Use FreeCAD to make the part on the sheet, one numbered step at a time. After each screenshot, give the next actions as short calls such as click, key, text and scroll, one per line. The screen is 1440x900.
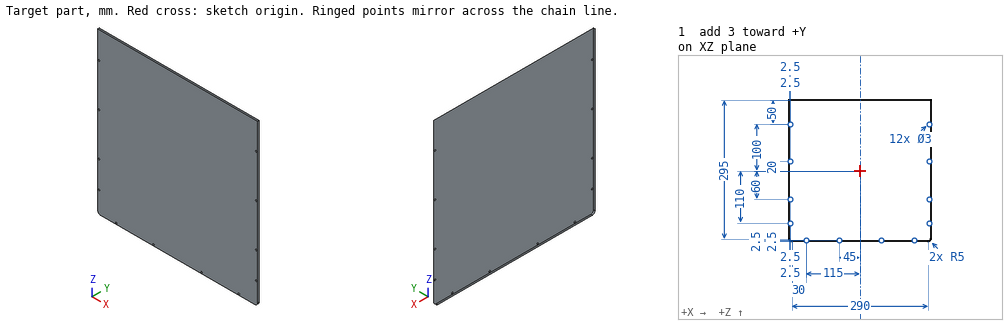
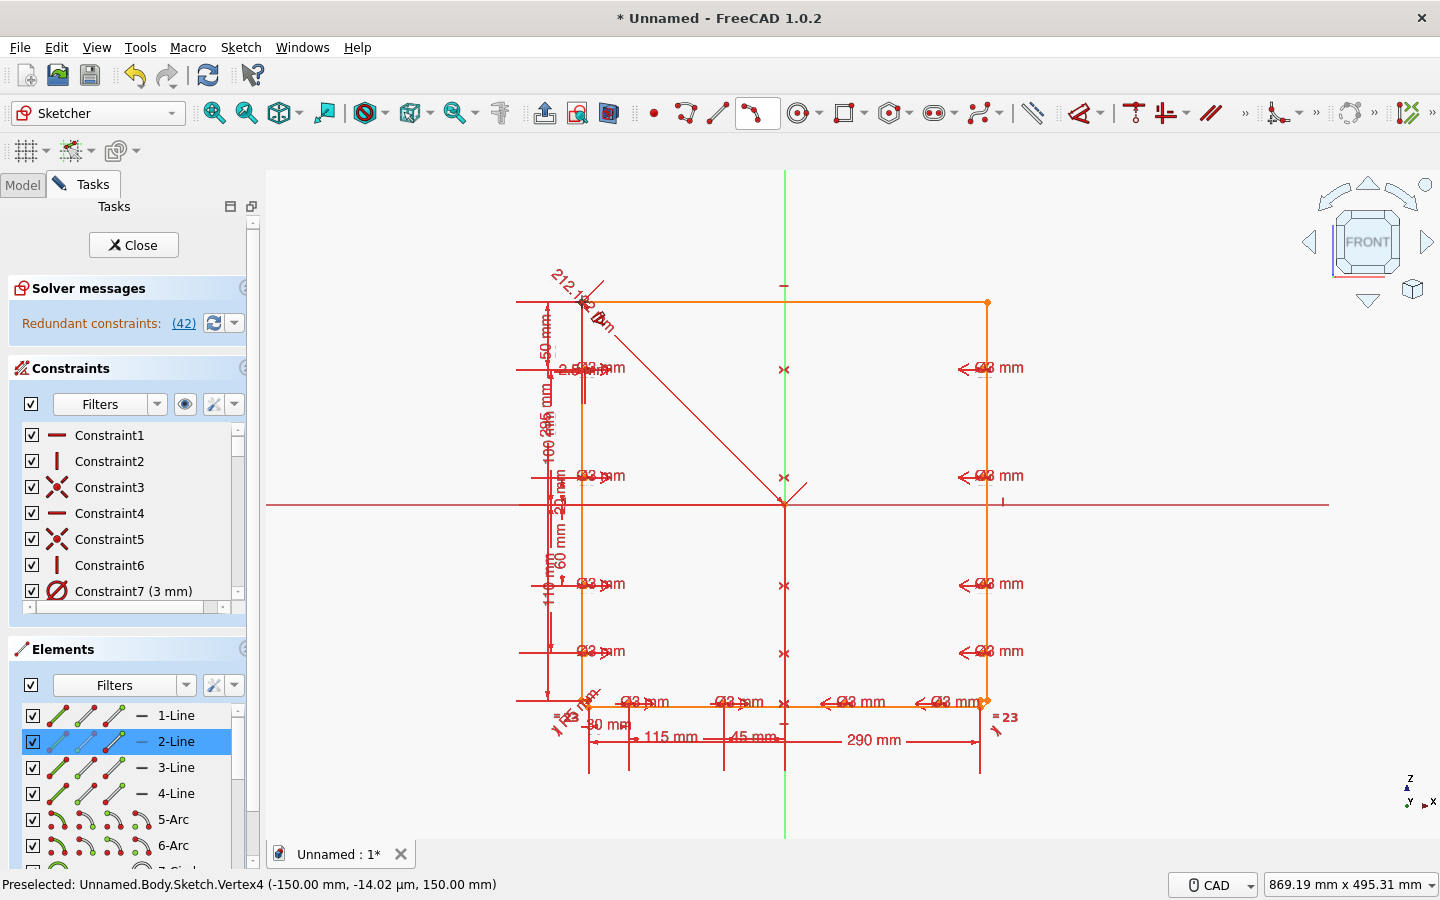
scroll(585, 478, up, 13)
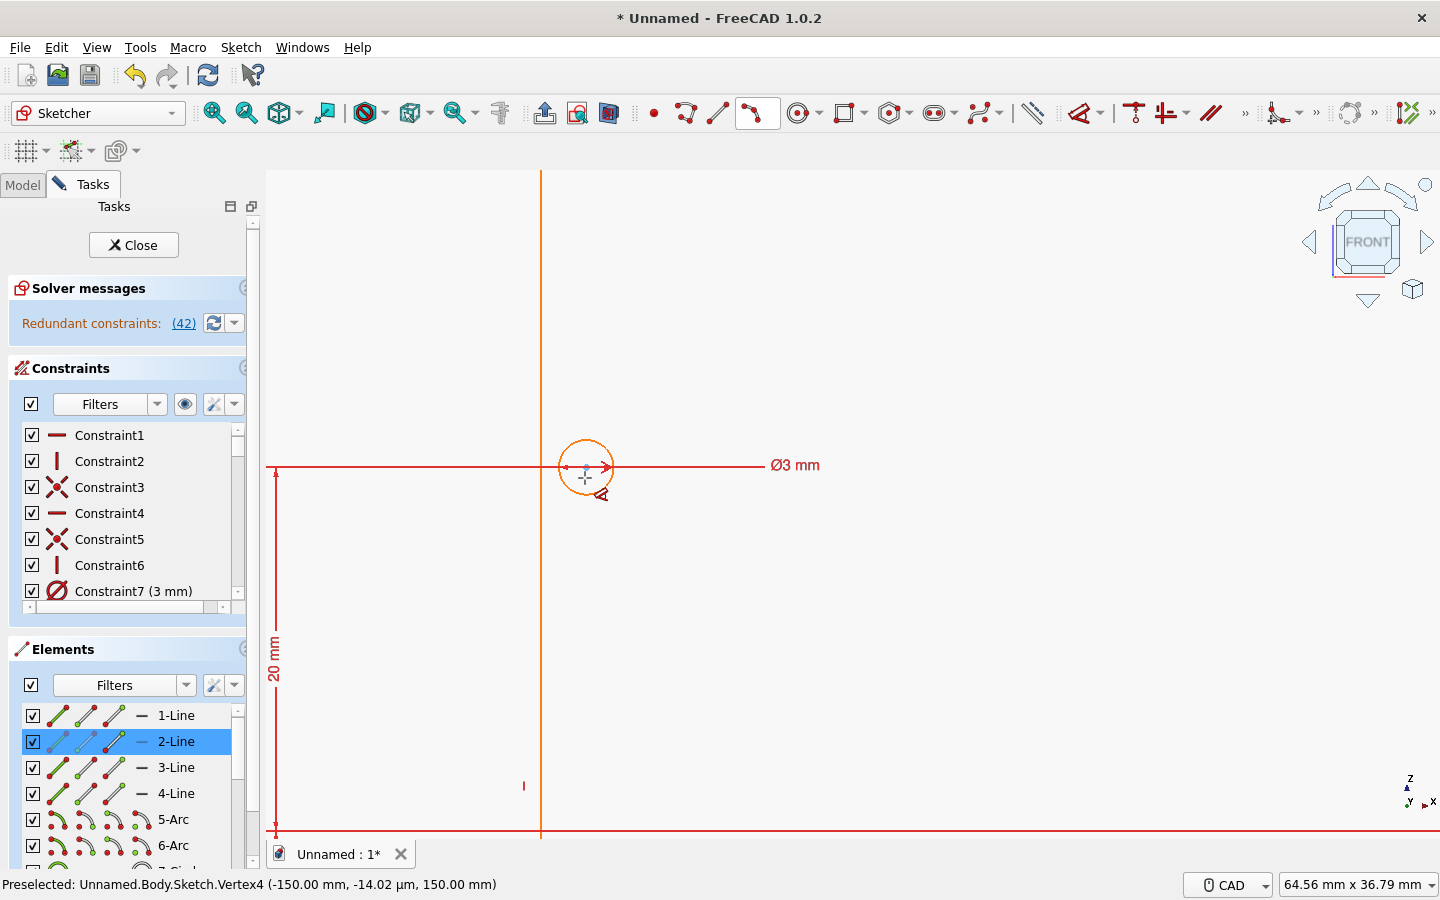
click(586, 467)
click(564, 501)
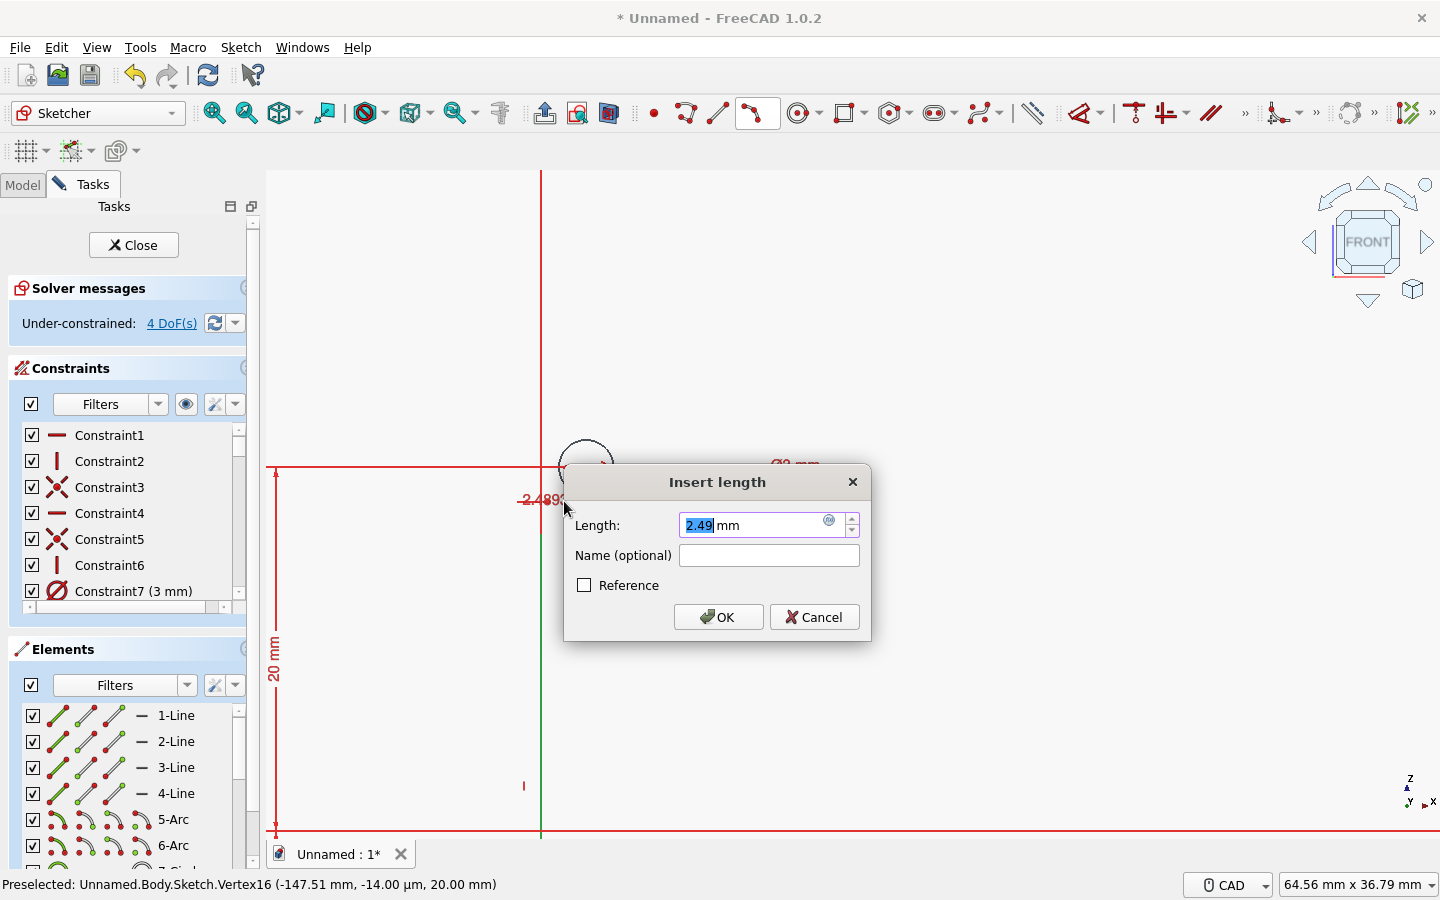
text(2.5)
key(Return)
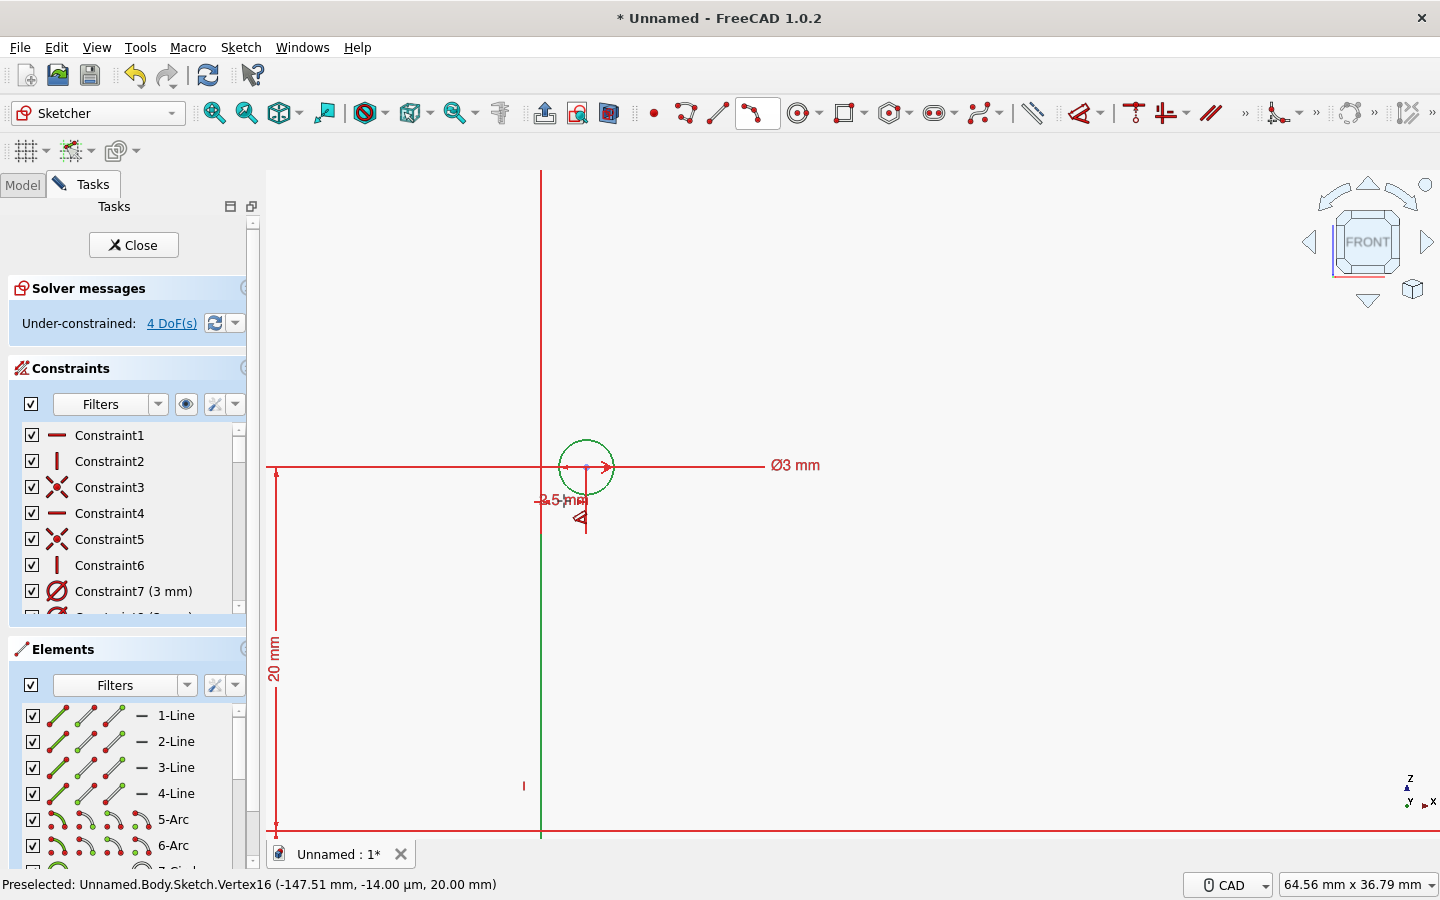
scroll(585, 478, down, 13)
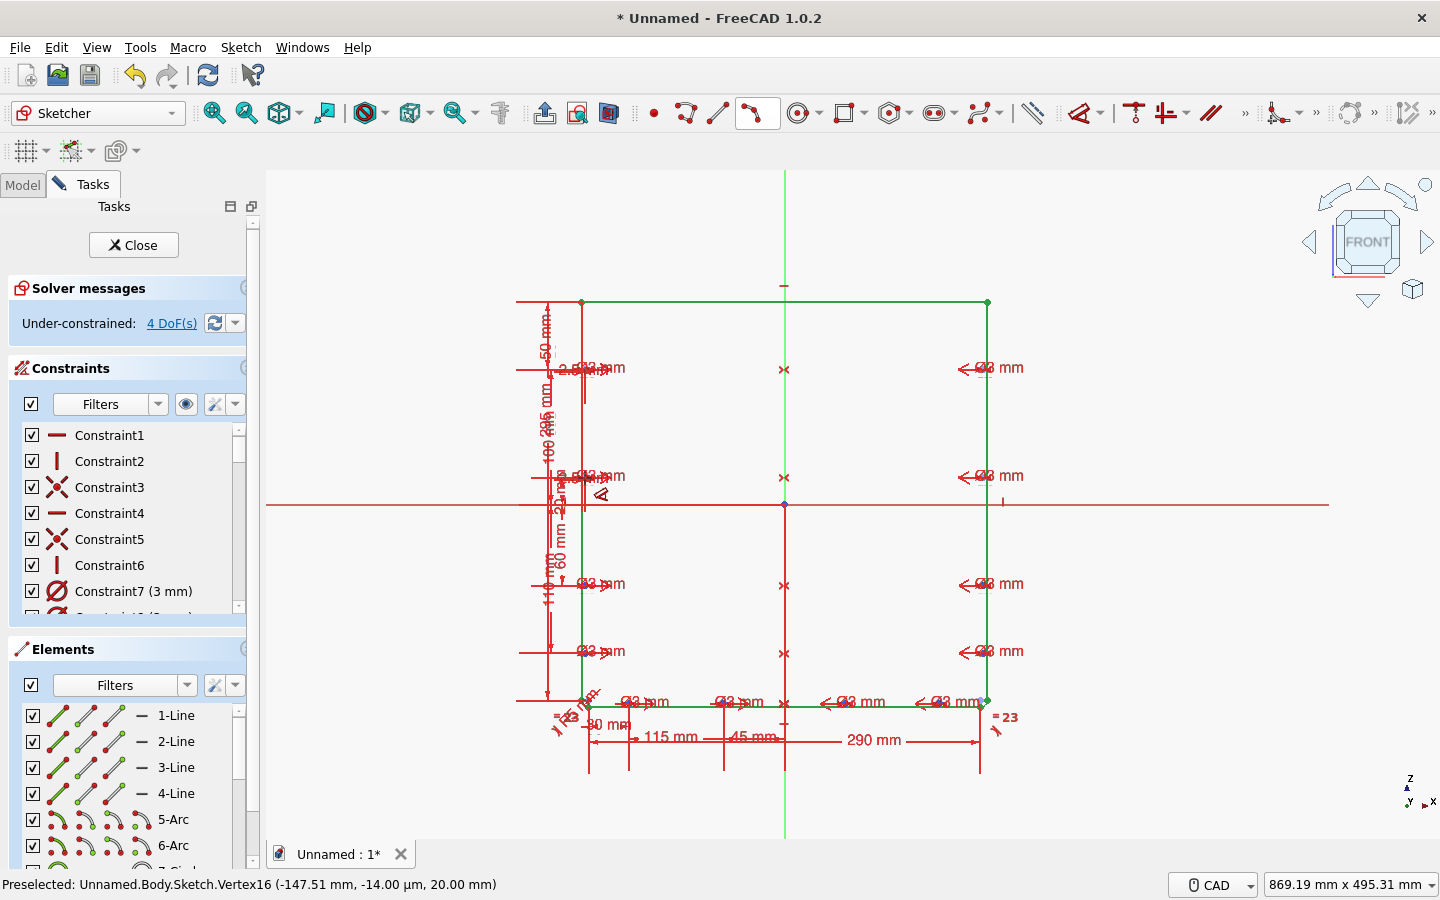
scroll(582, 700, up, 13)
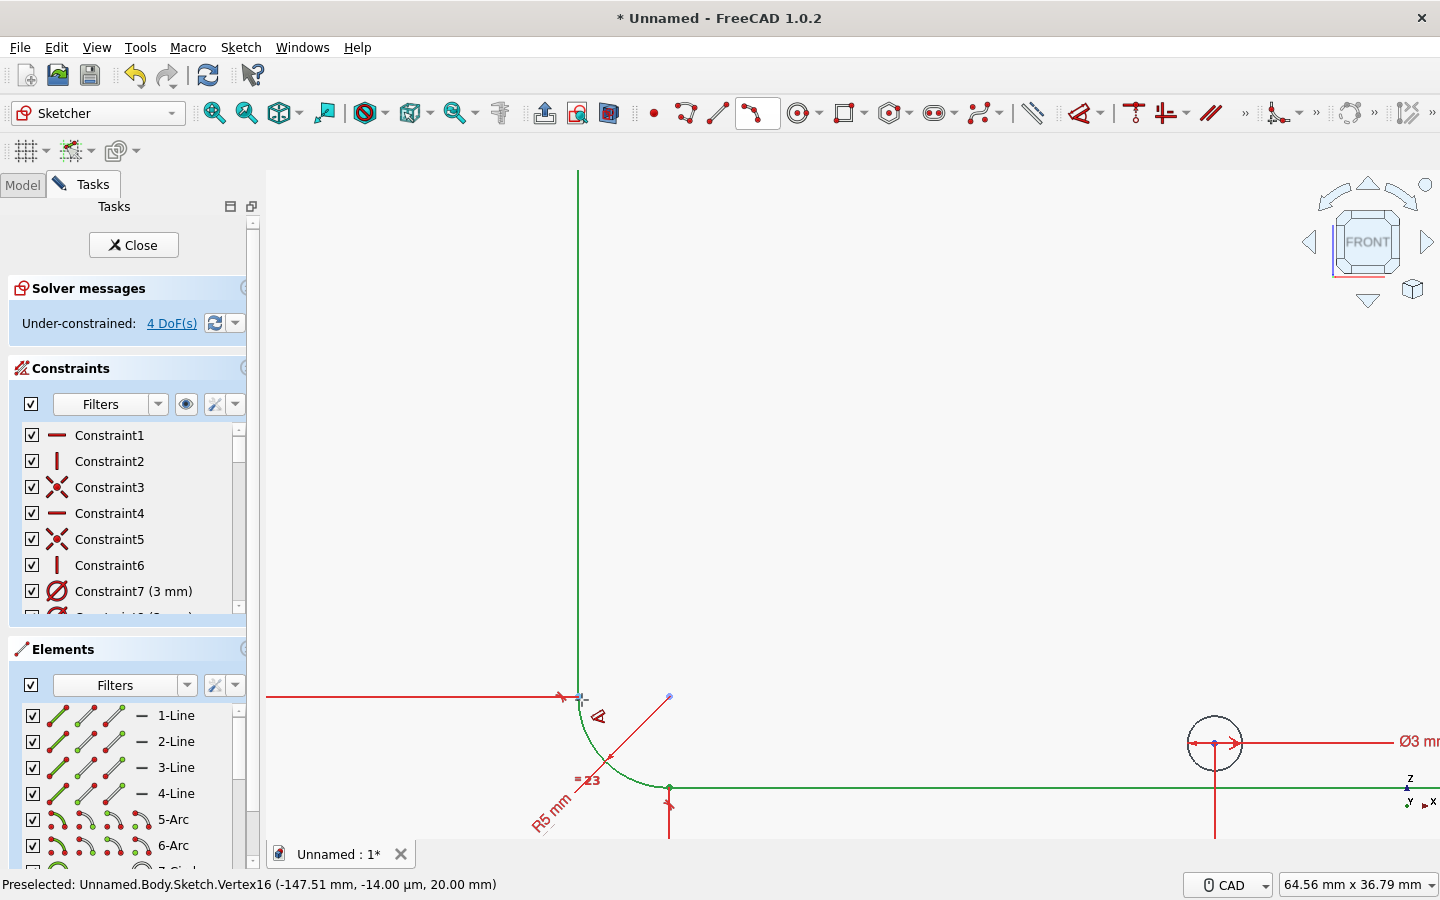
click(578, 697)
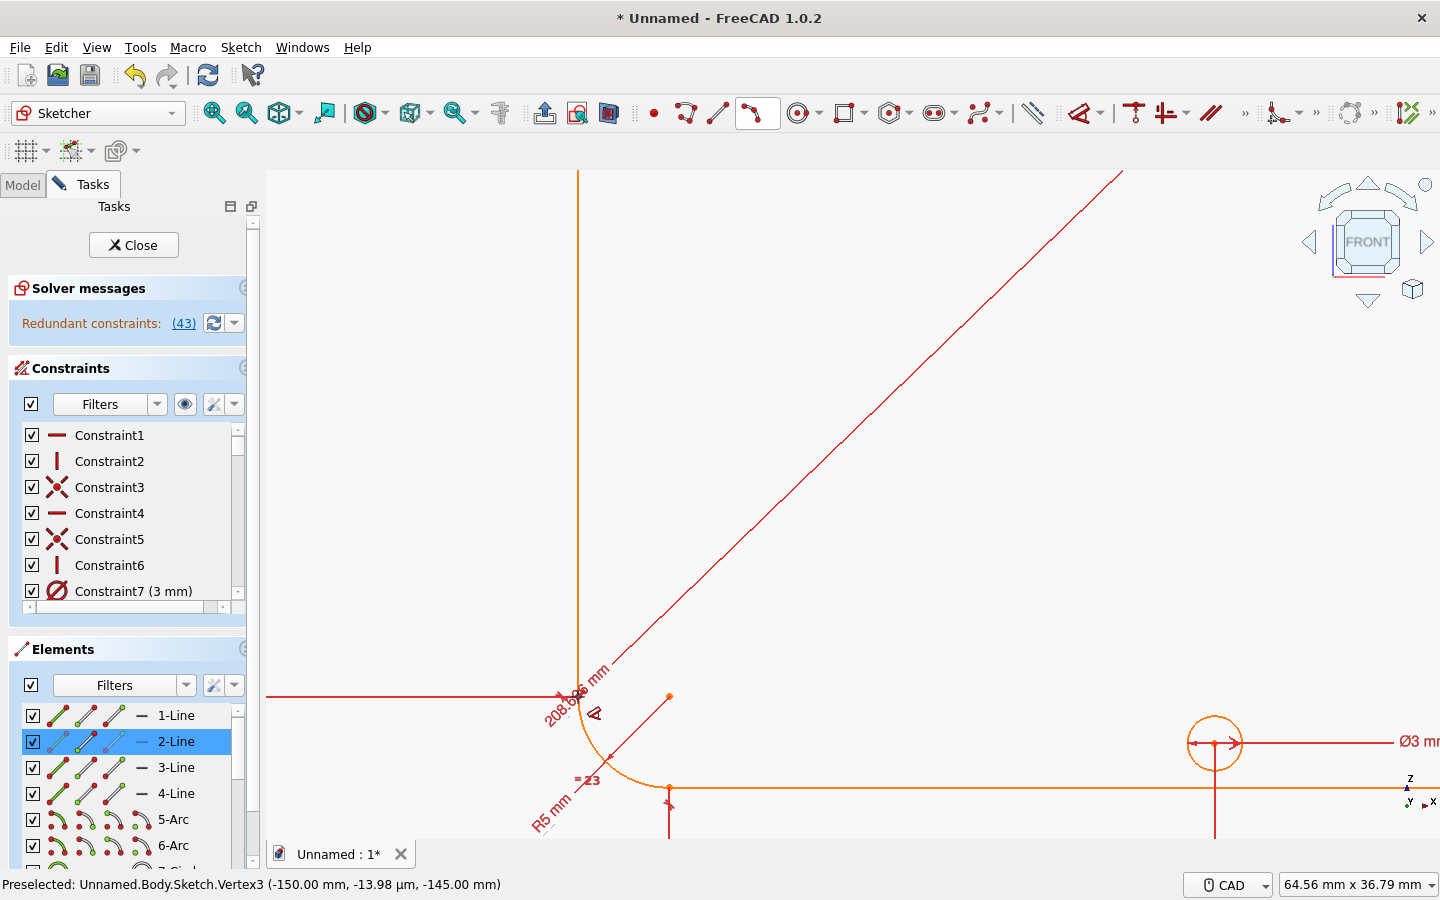
scroll(582, 701, down, 13)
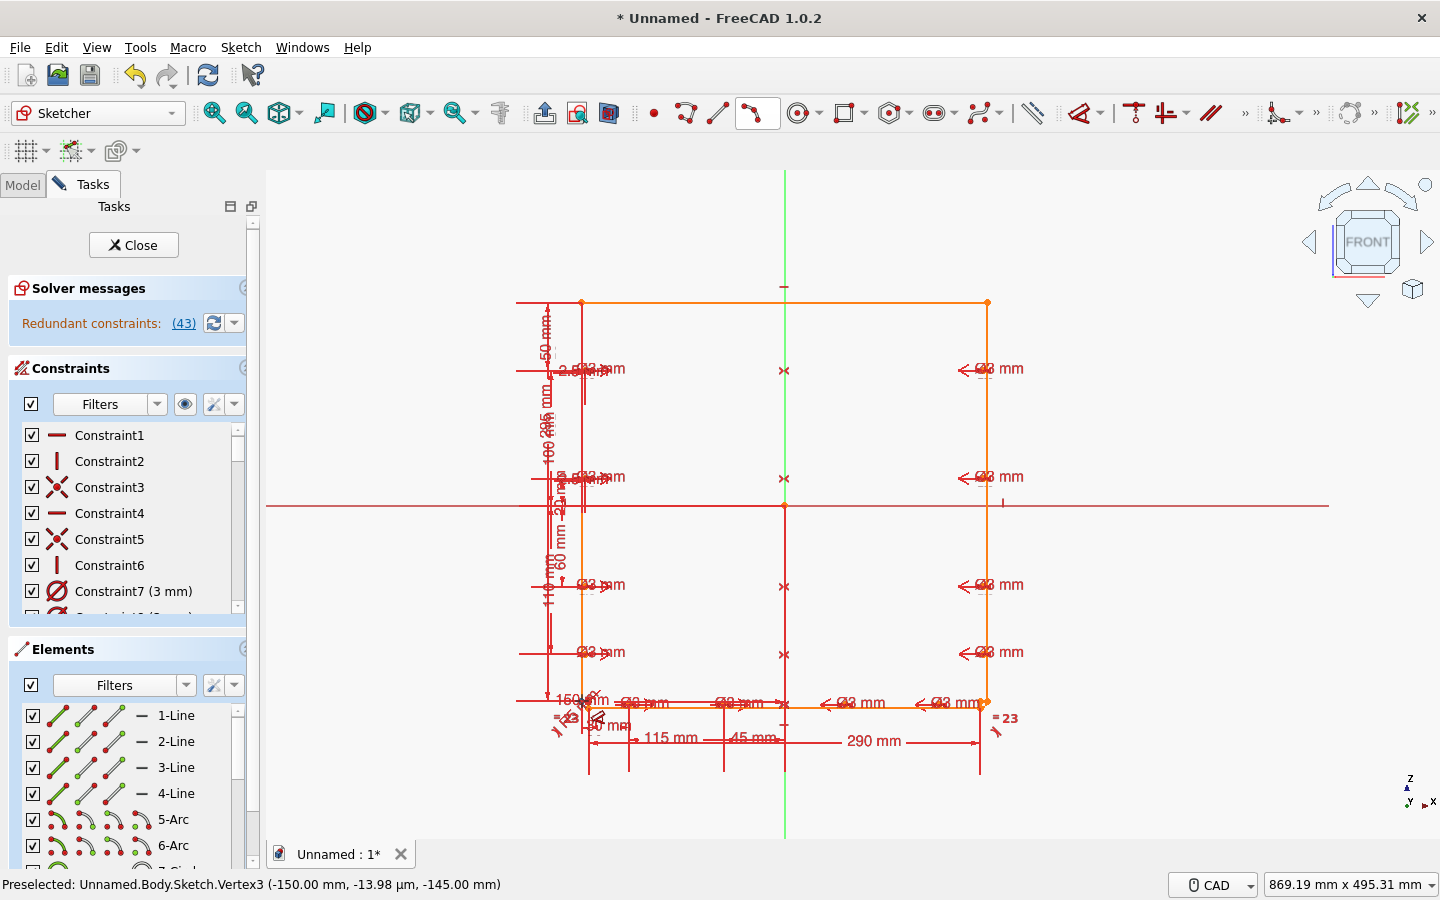
scroll(585, 587, up, 13)